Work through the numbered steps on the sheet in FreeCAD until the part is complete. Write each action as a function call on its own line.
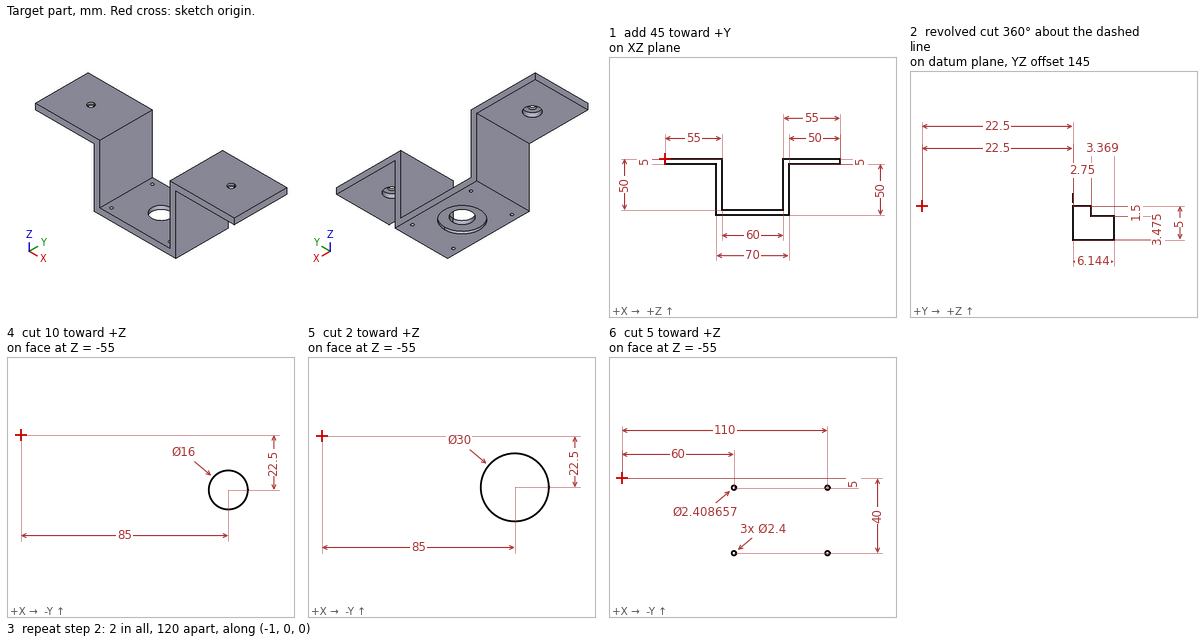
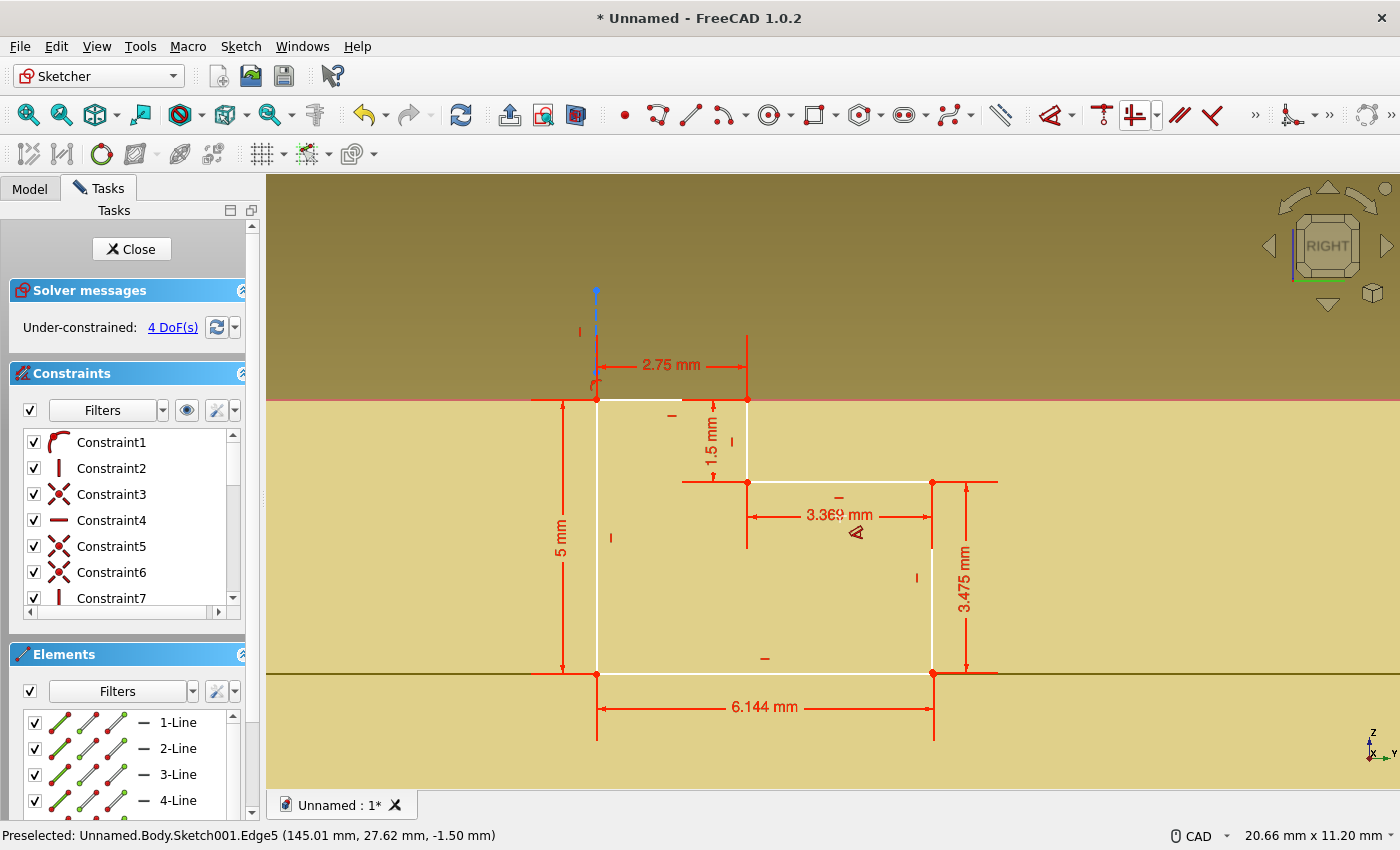
click(597, 400)
click(445, 366)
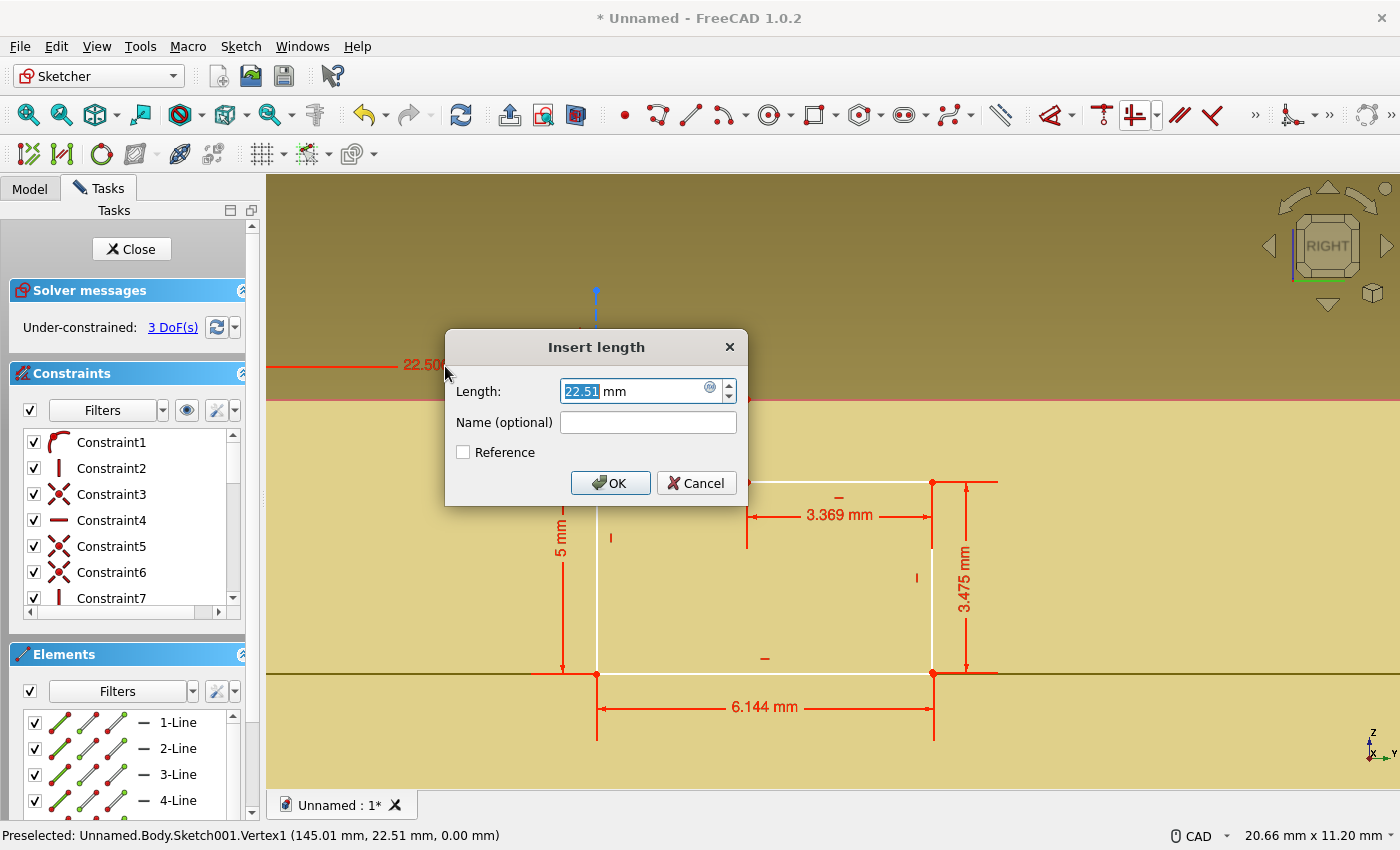
text(22.5)
key(Return)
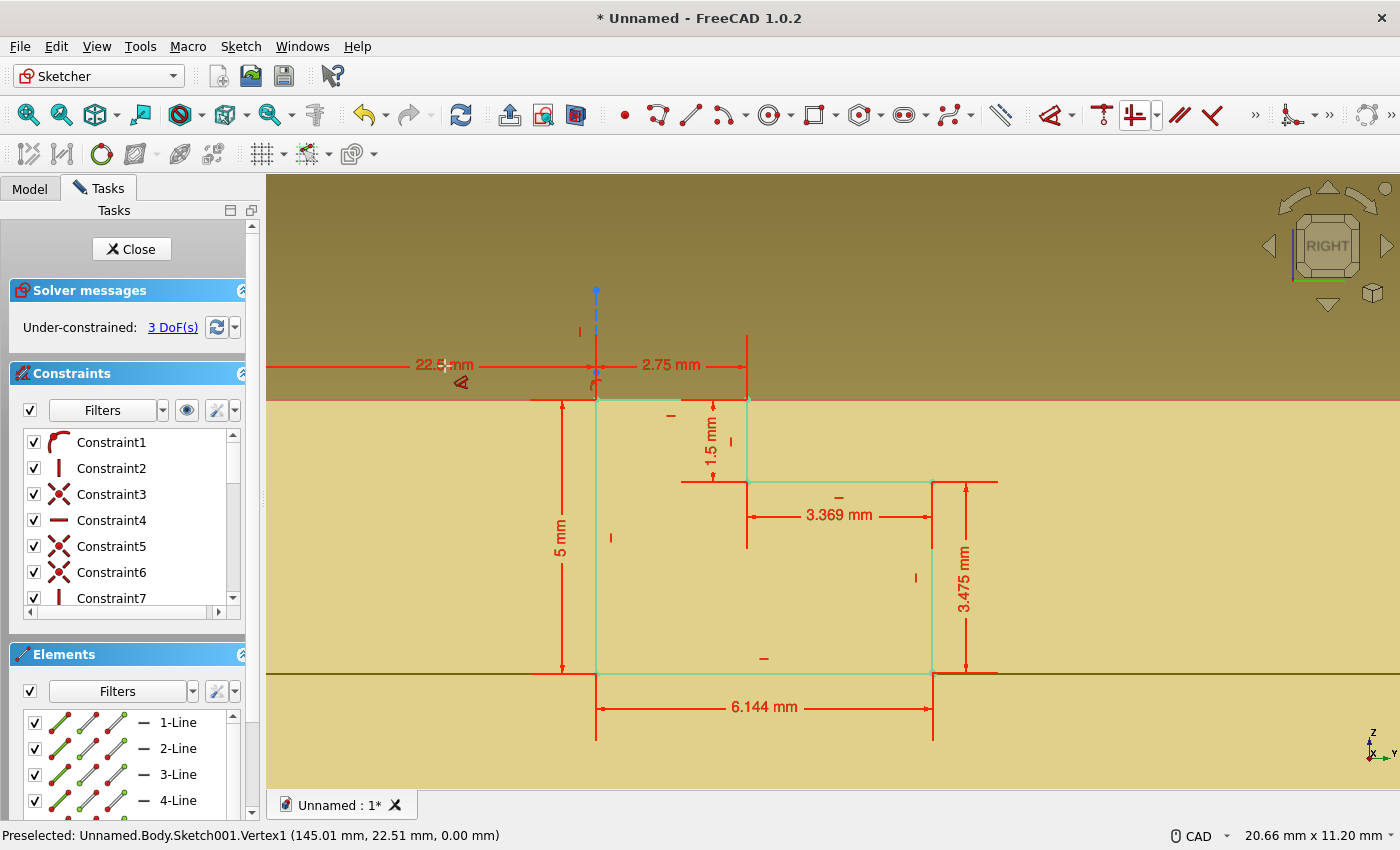
click(596, 373)
click(445, 339)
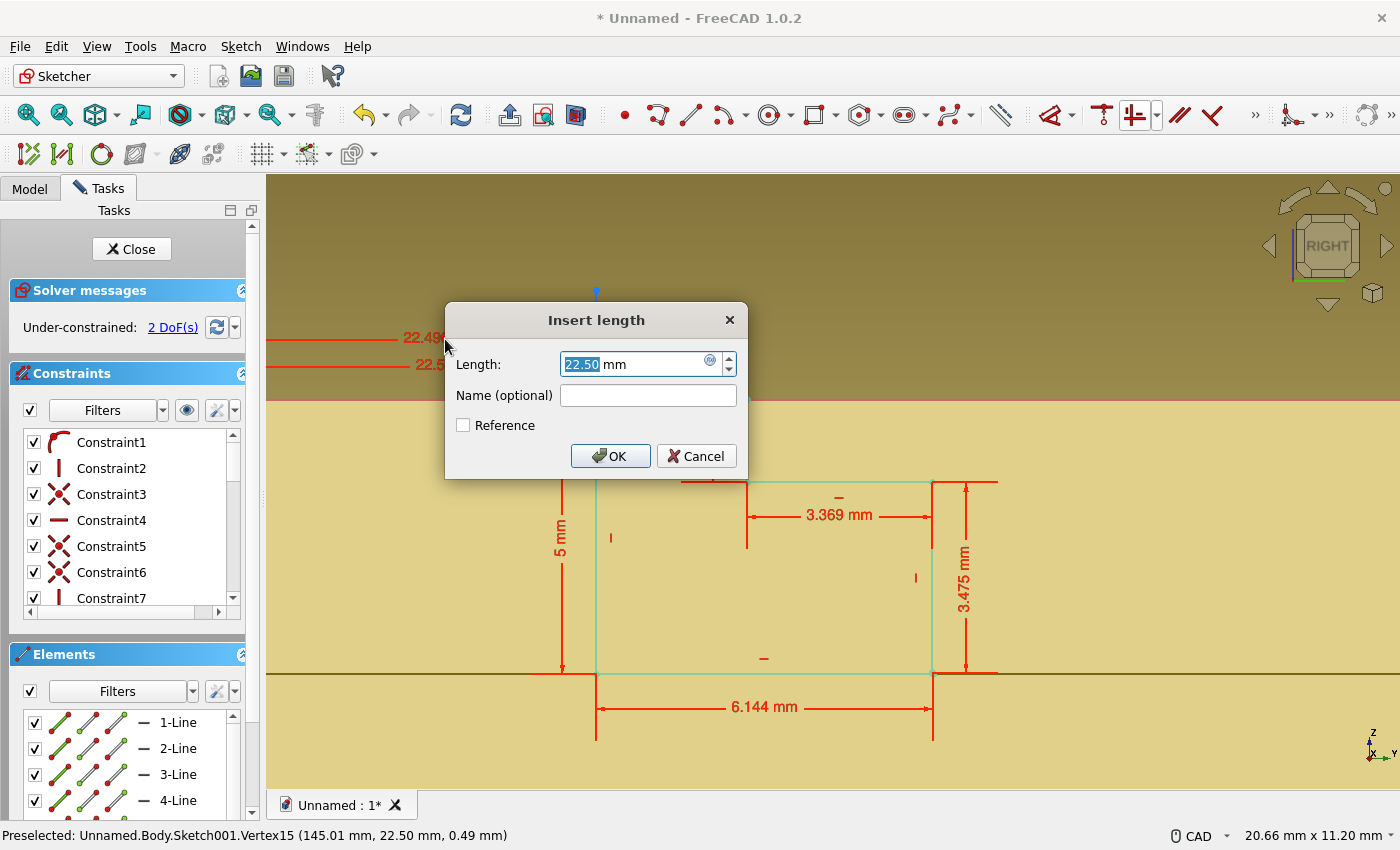
text(22.5)
key(Return)
key(Escape)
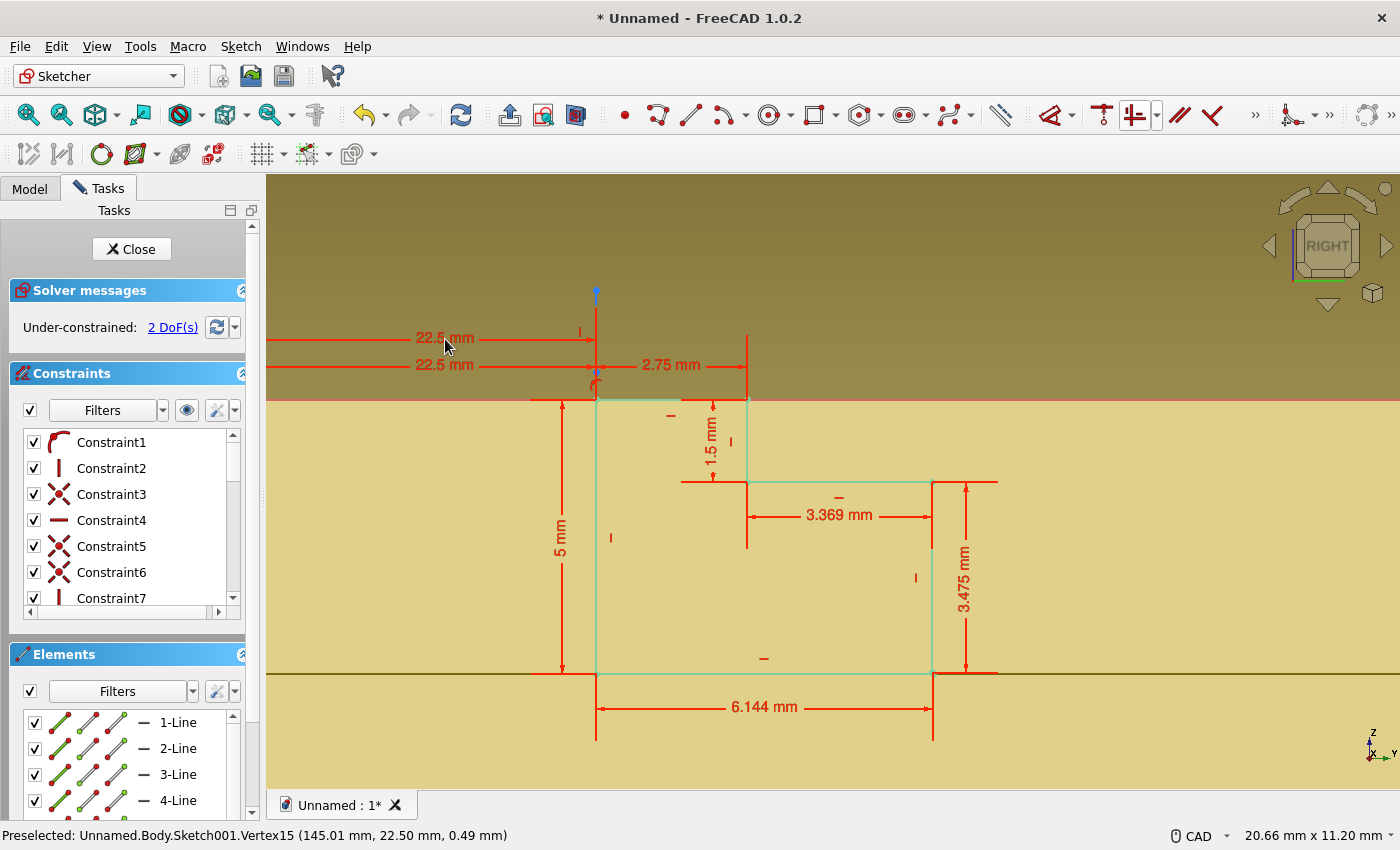
click(132, 249)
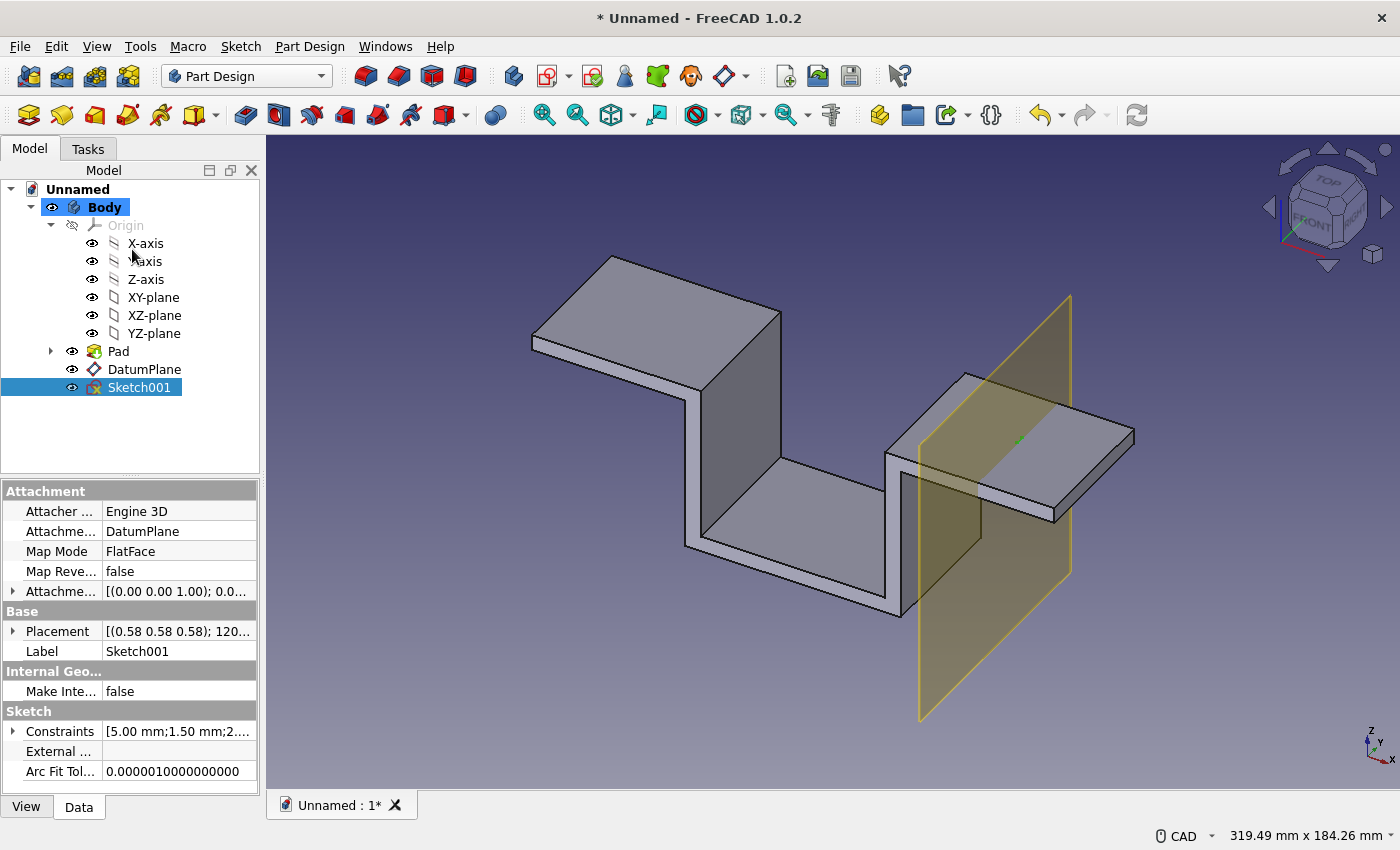
click(312, 116)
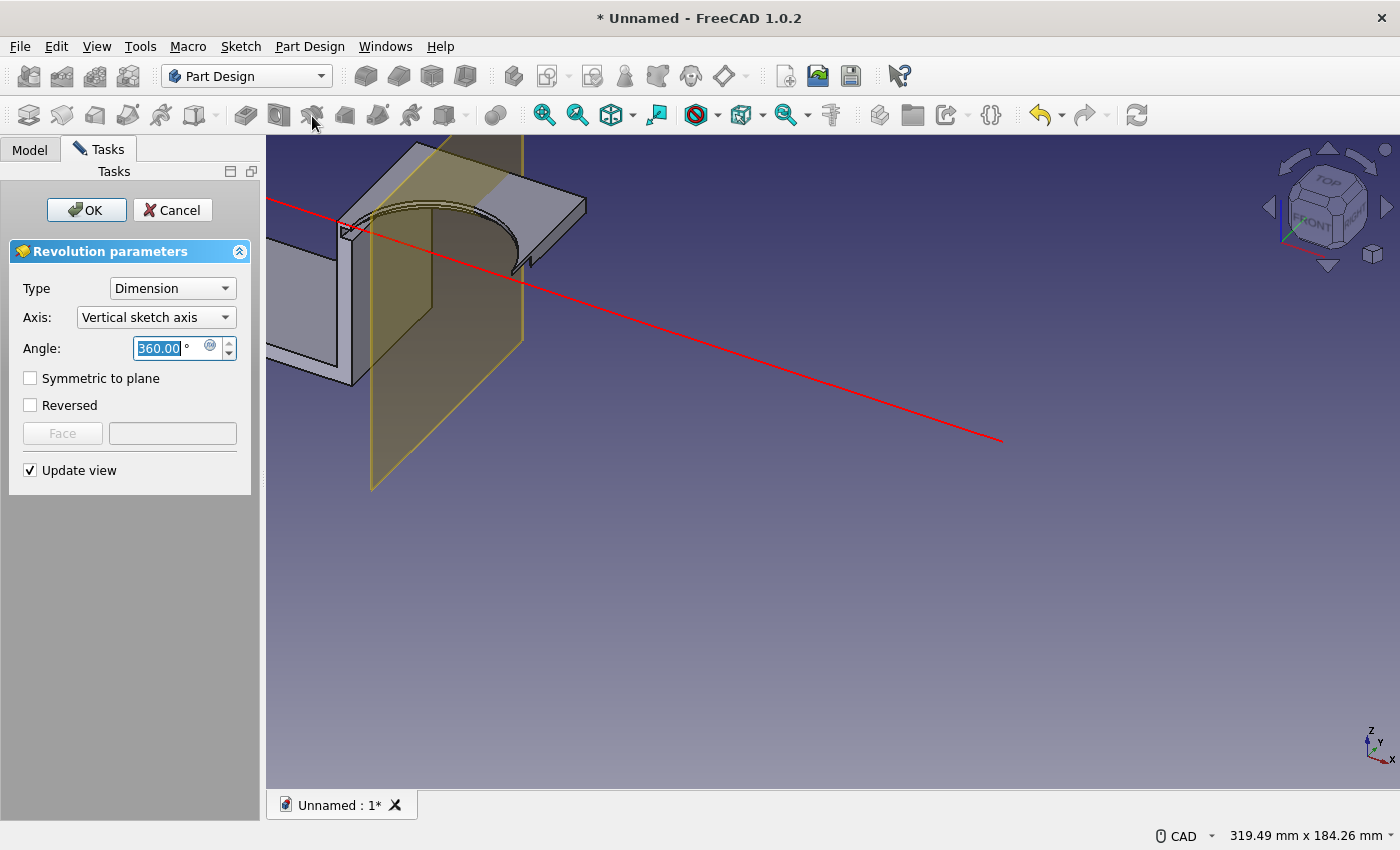
click(157, 318)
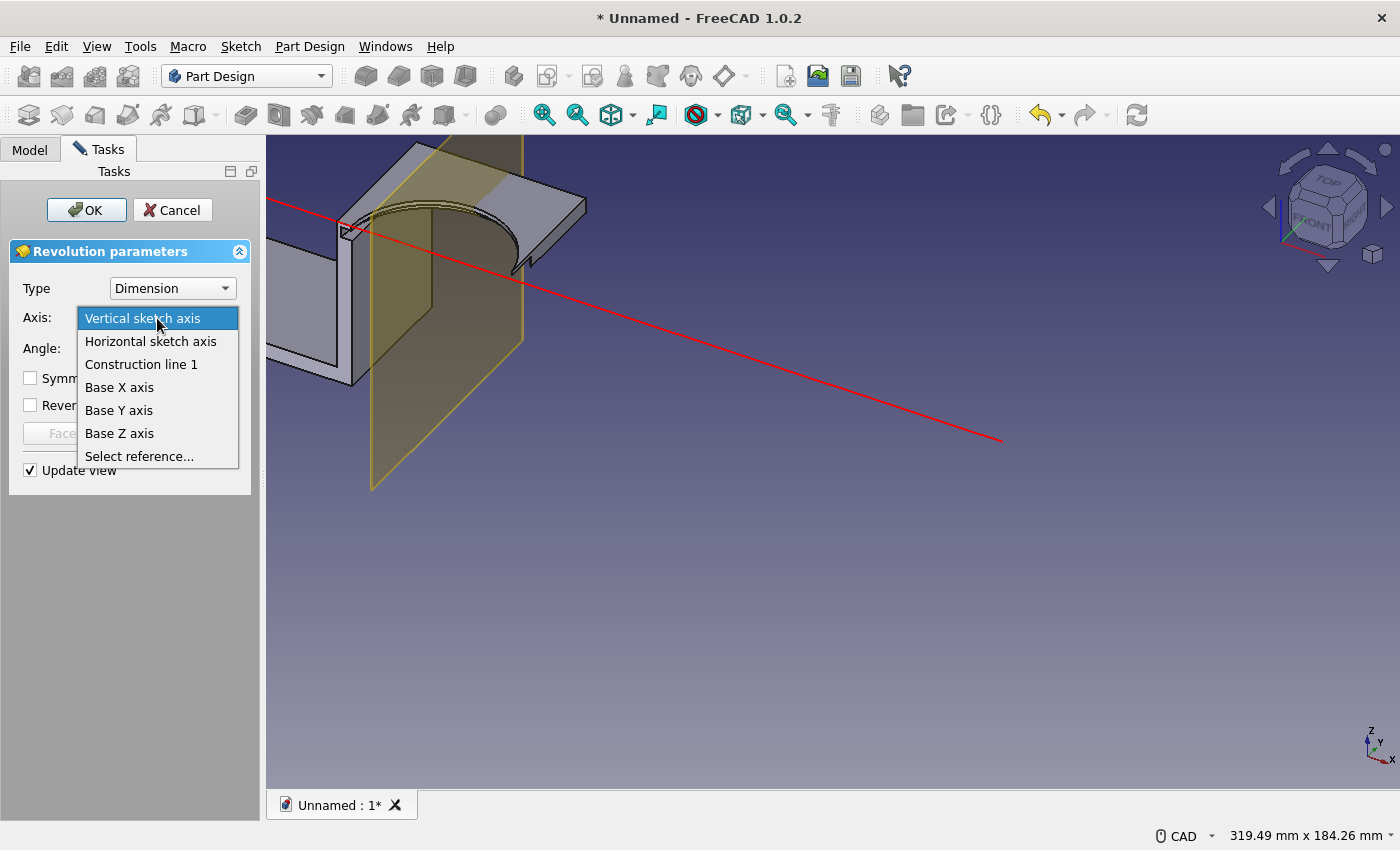
click(156, 364)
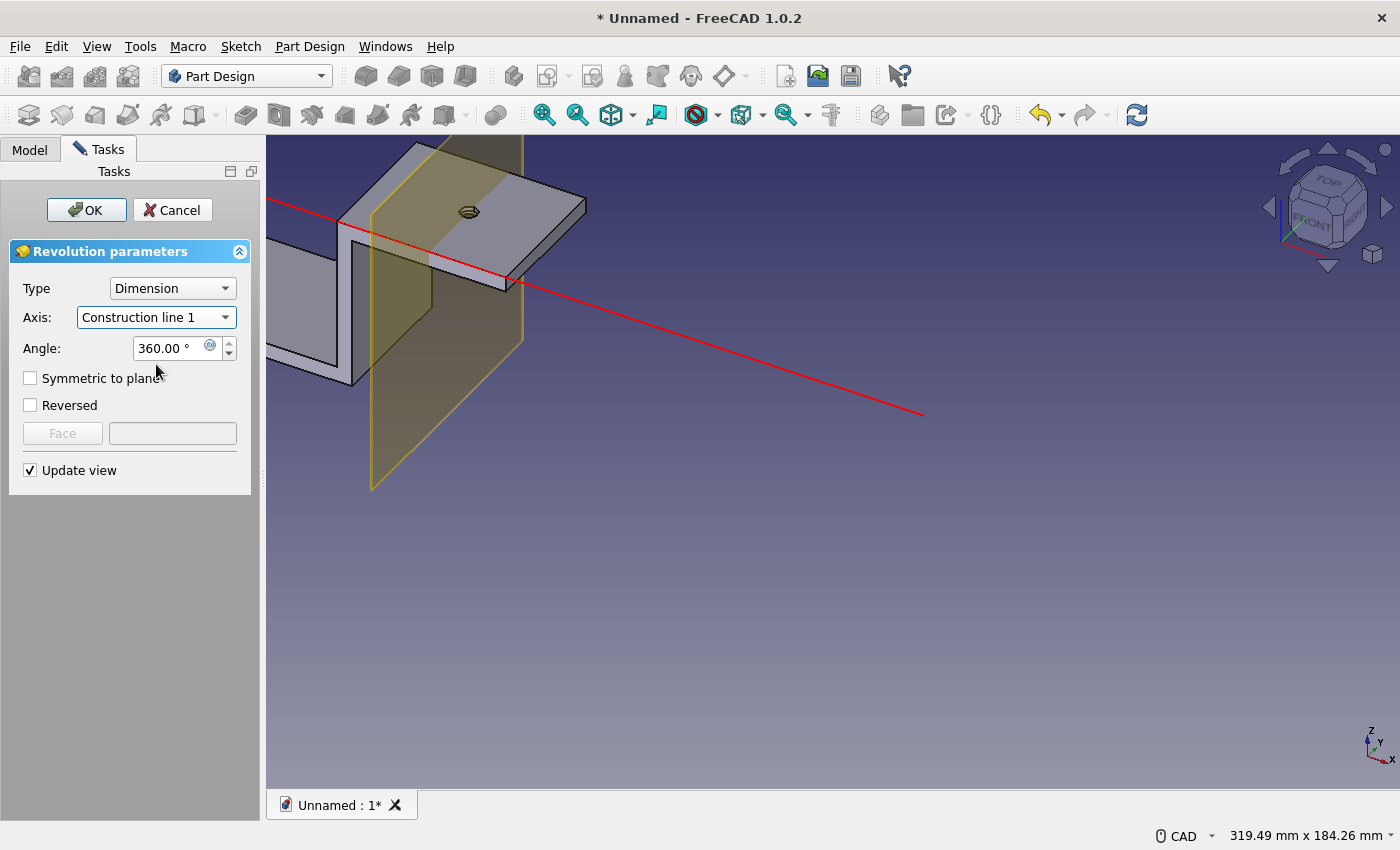
click(87, 210)